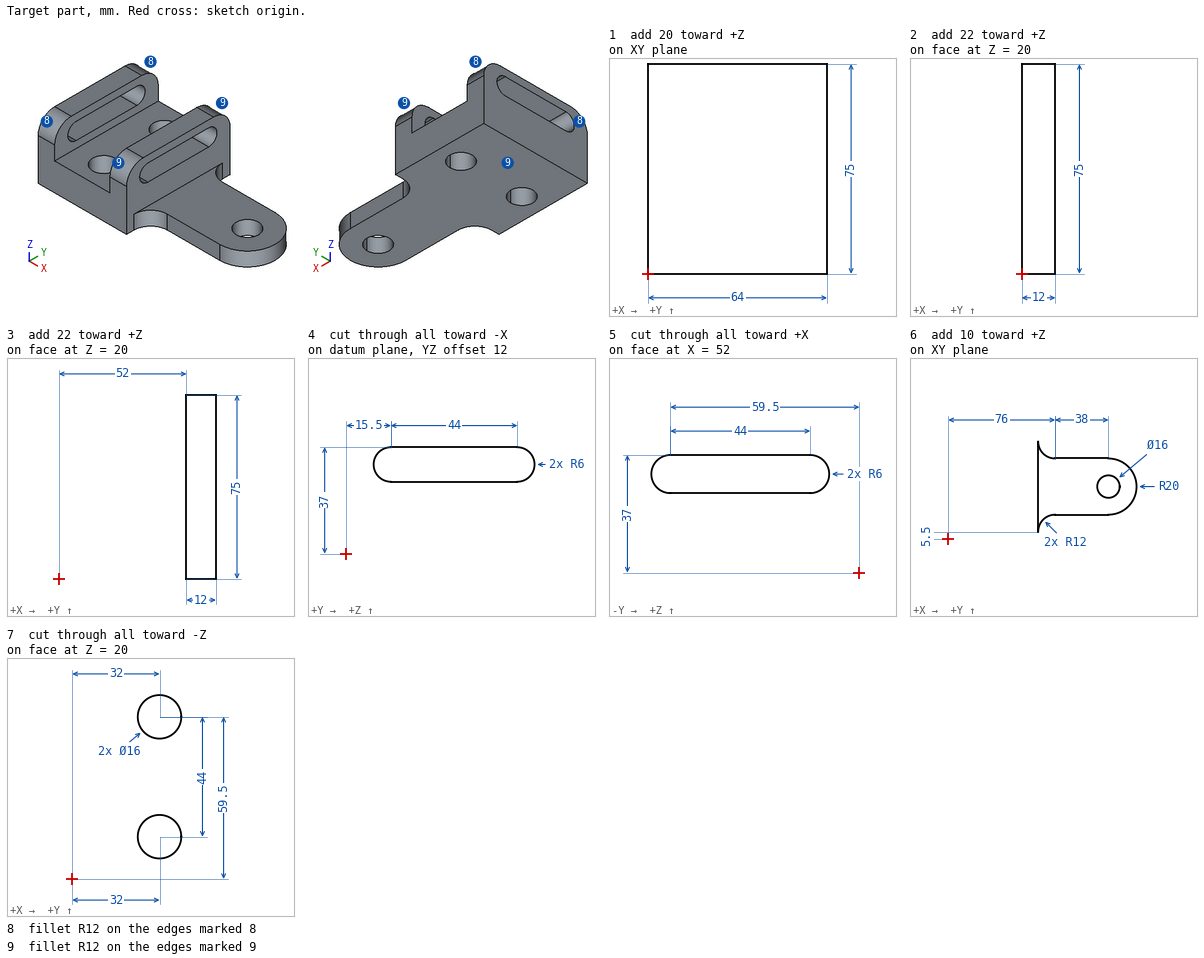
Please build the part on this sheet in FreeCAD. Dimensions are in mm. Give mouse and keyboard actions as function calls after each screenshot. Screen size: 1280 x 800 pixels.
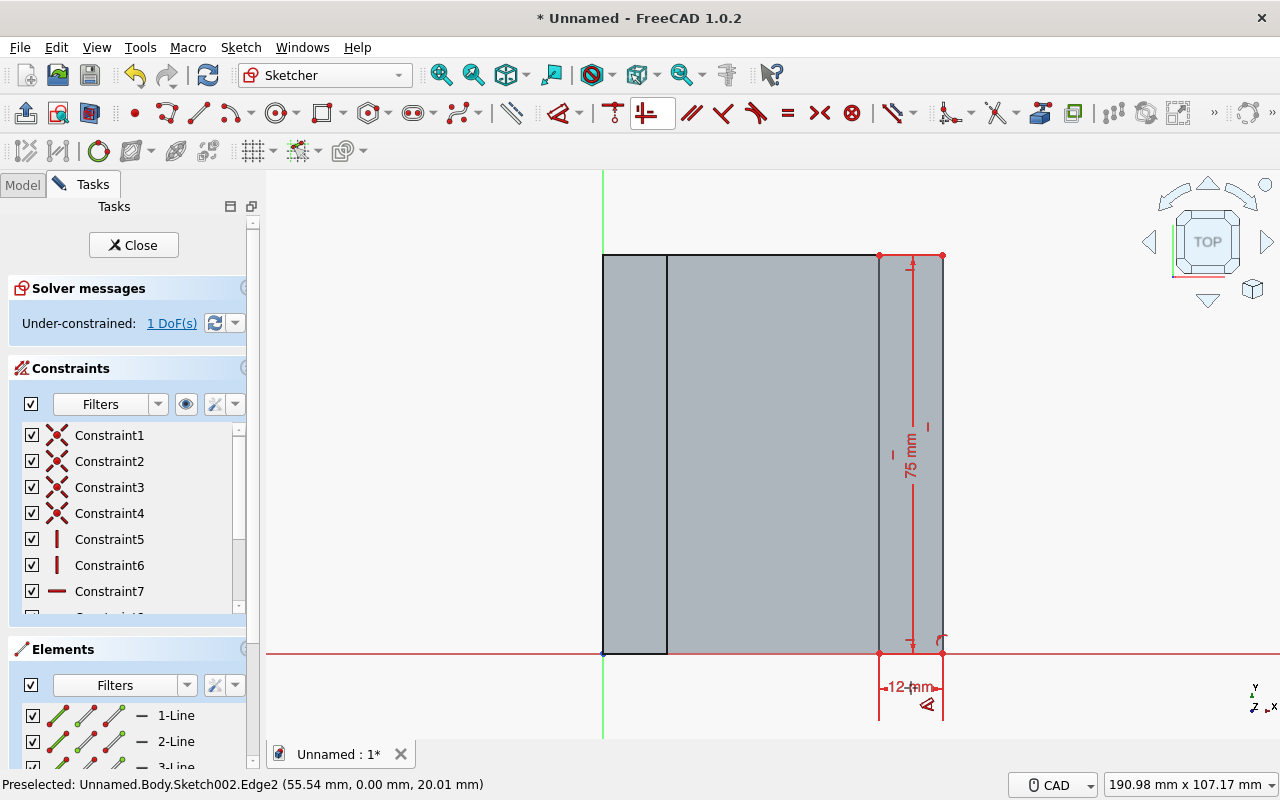
click(879, 255)
click(741, 688)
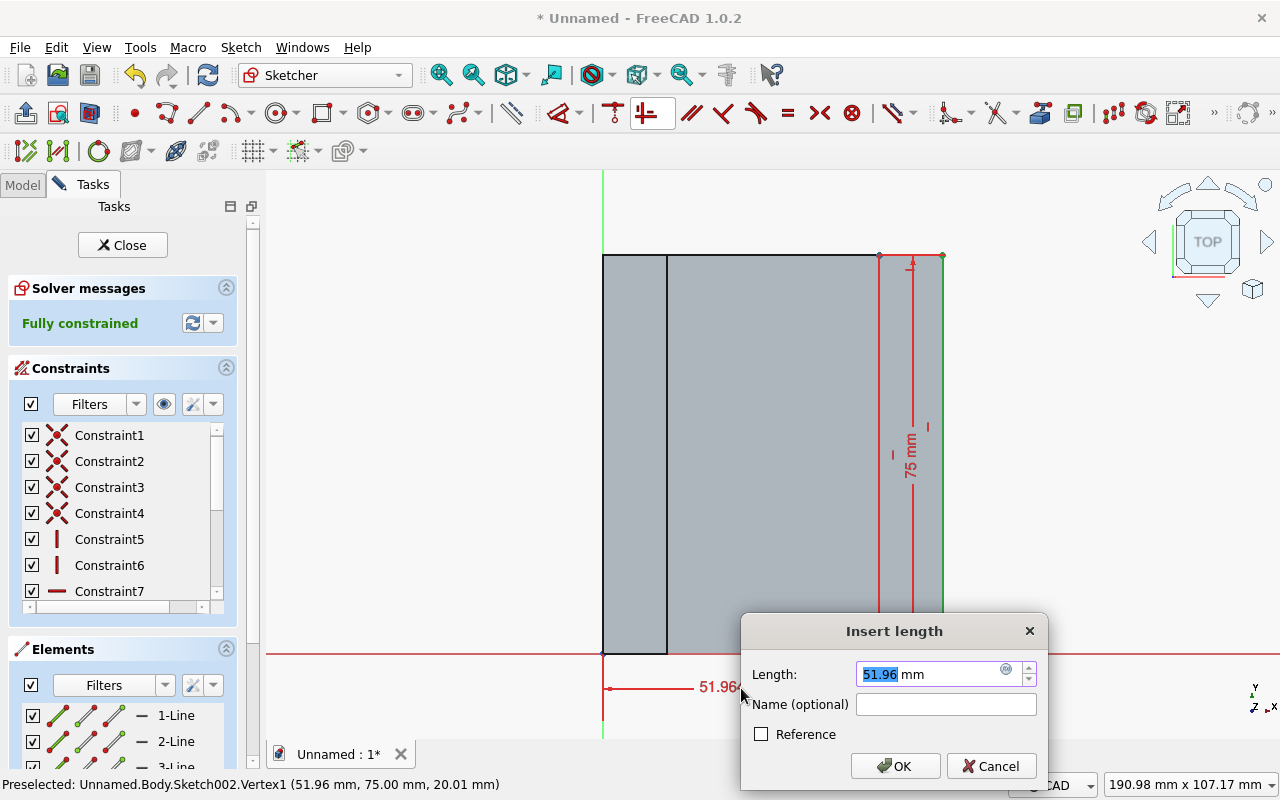
text(52)
key(Return)
key(Escape)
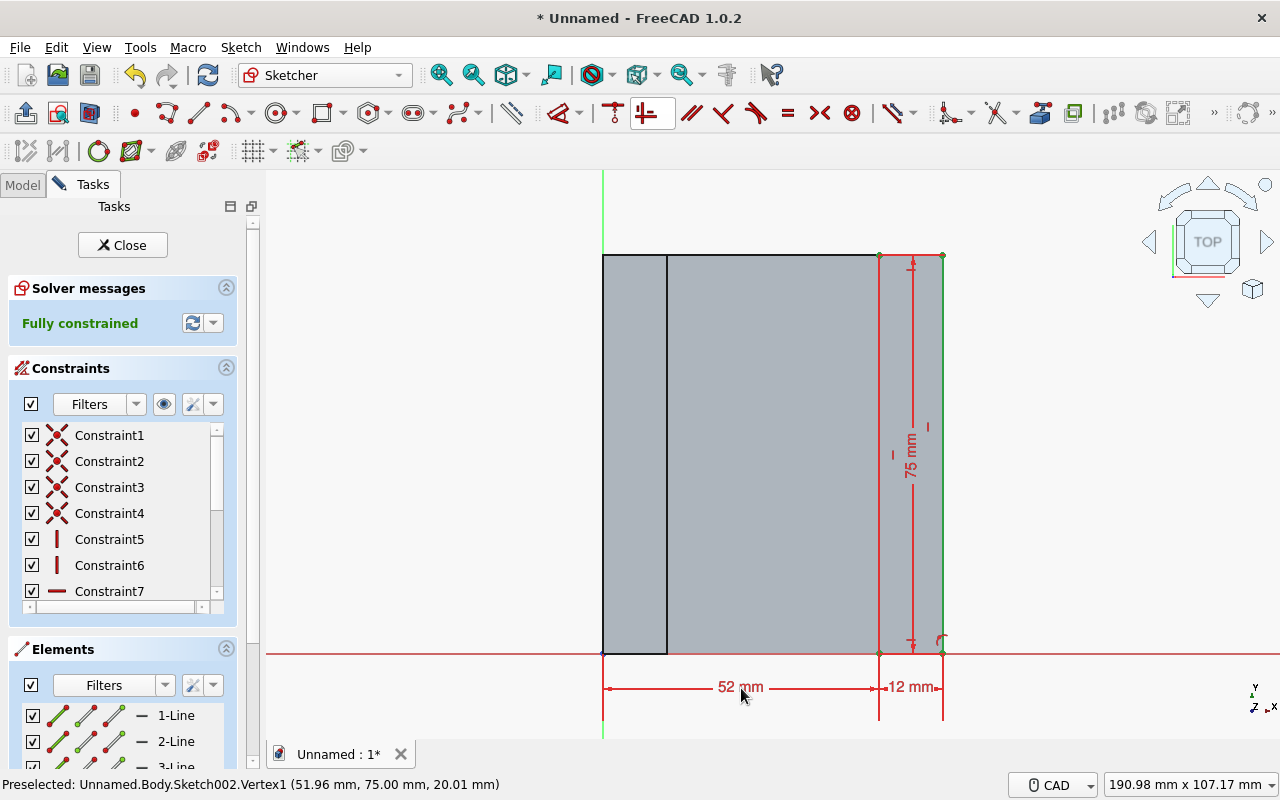
click(123, 245)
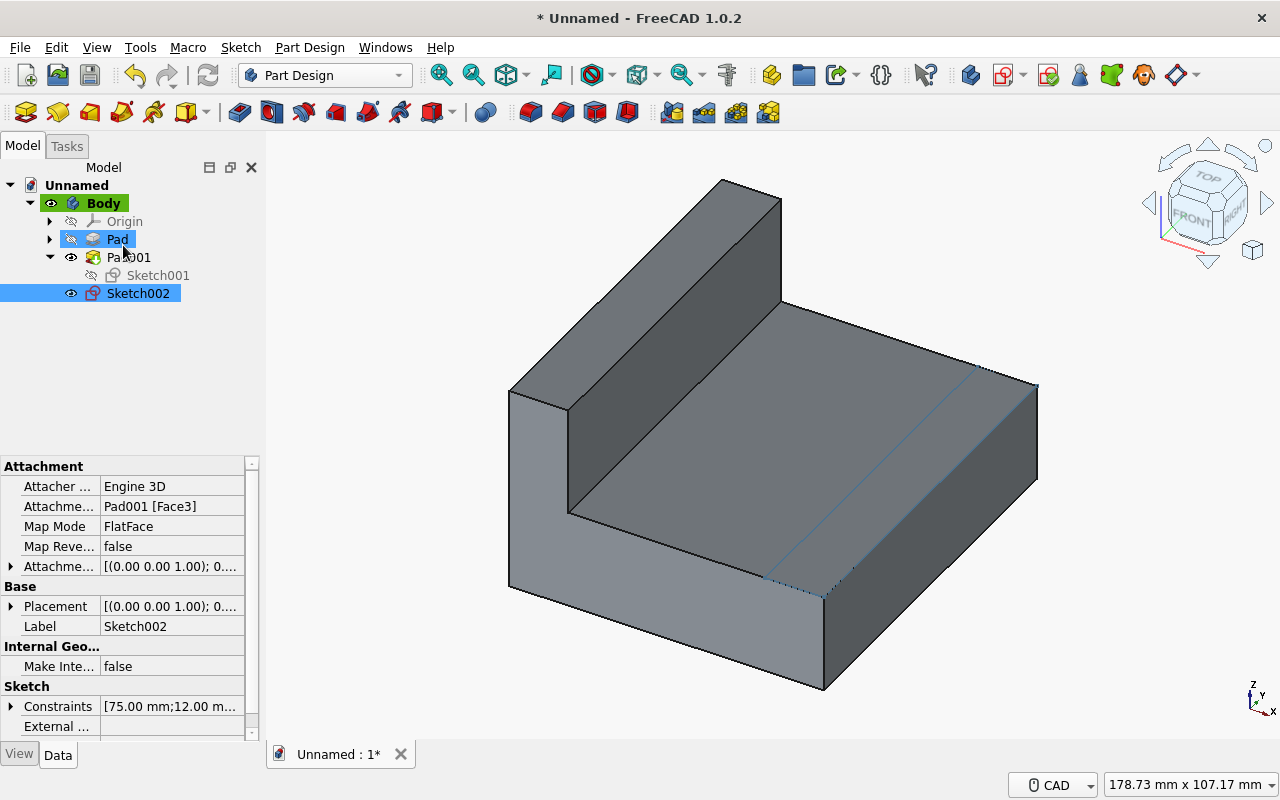
click(26, 112)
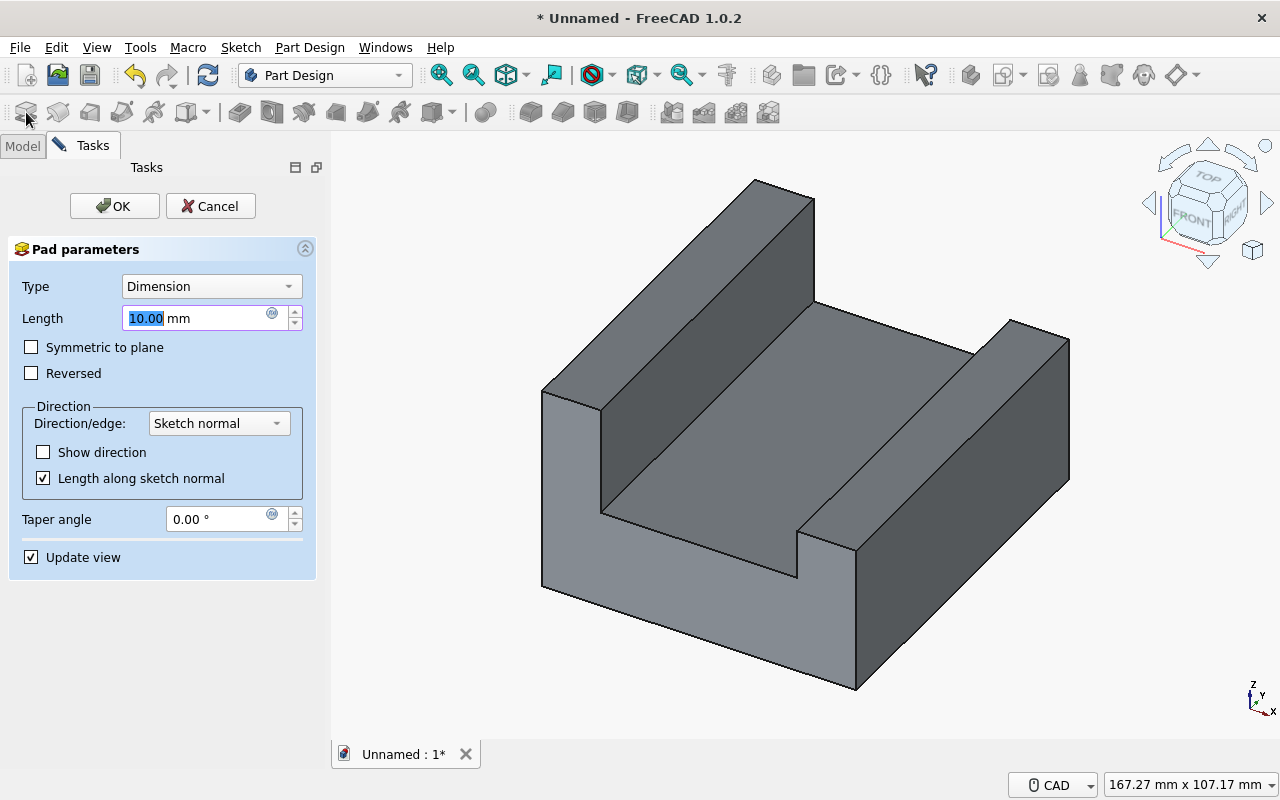
text(22)
key(Tab)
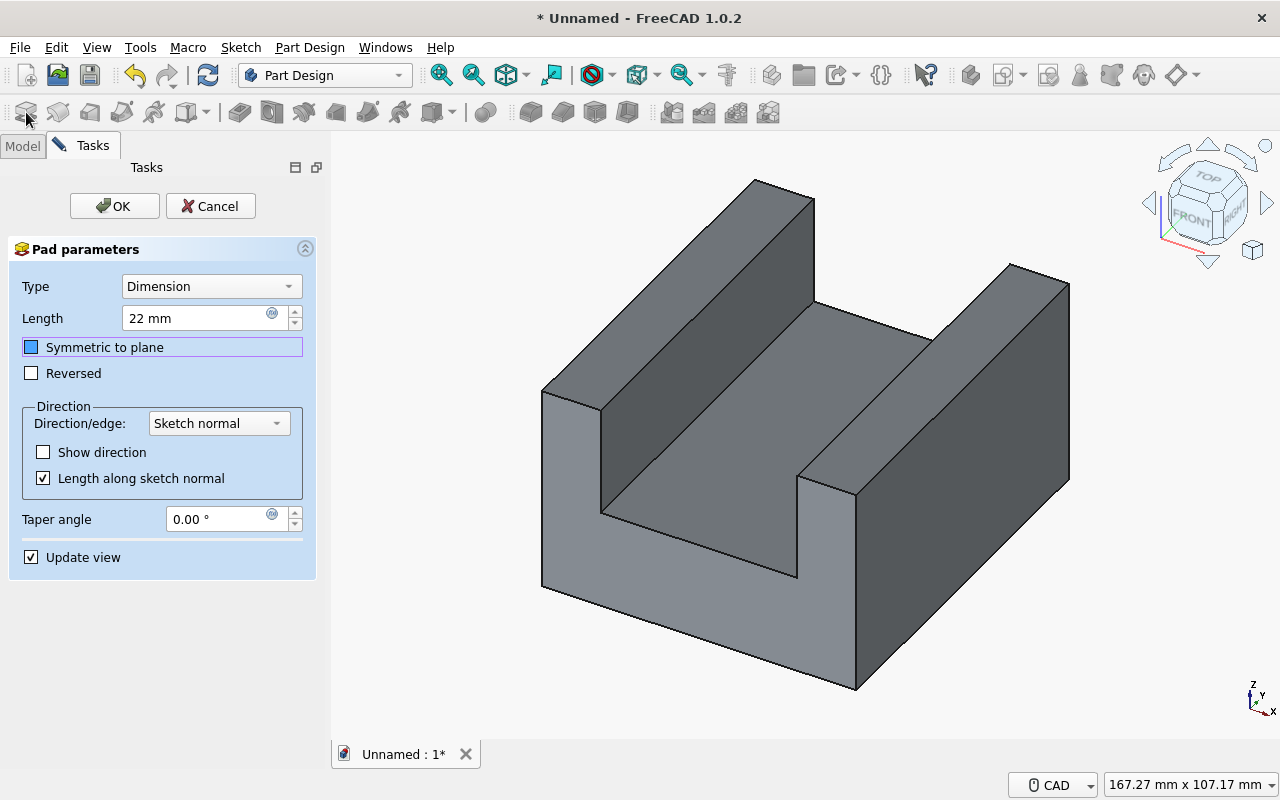
click(115, 206)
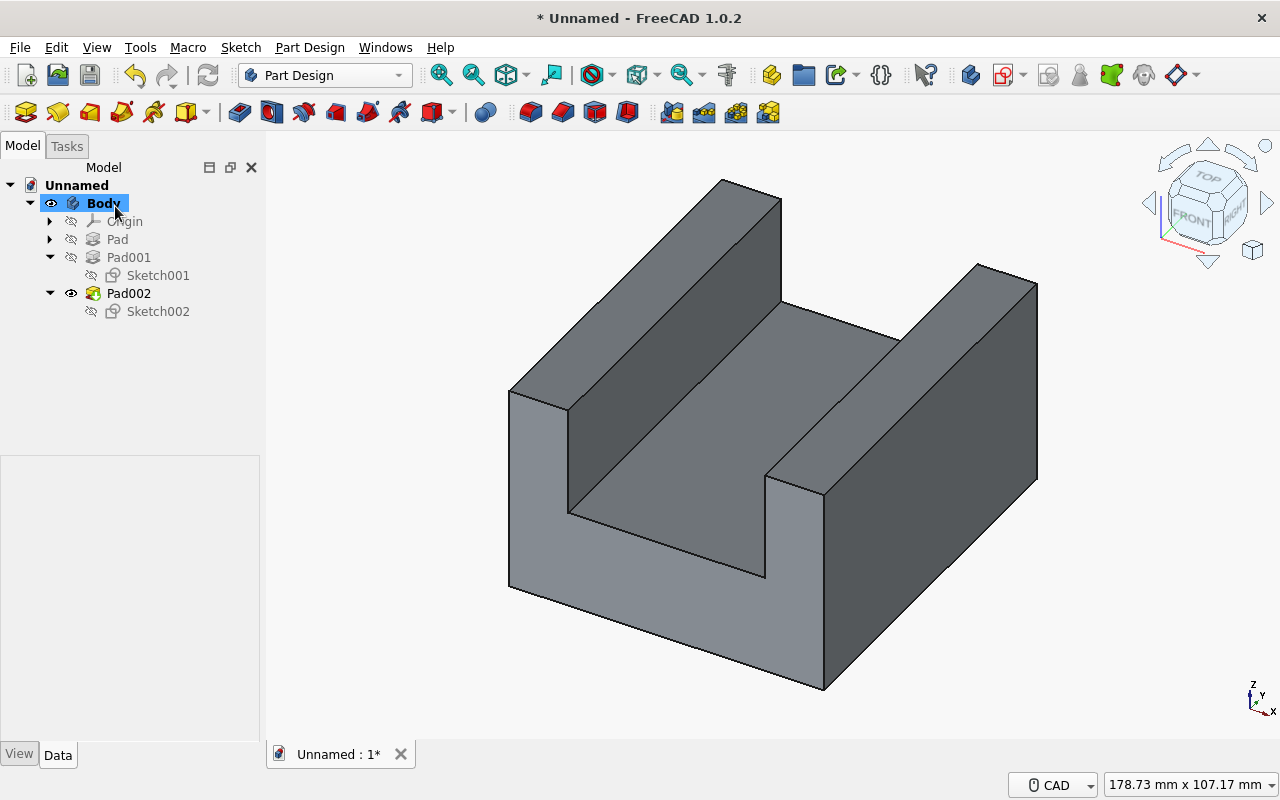
click(50, 221)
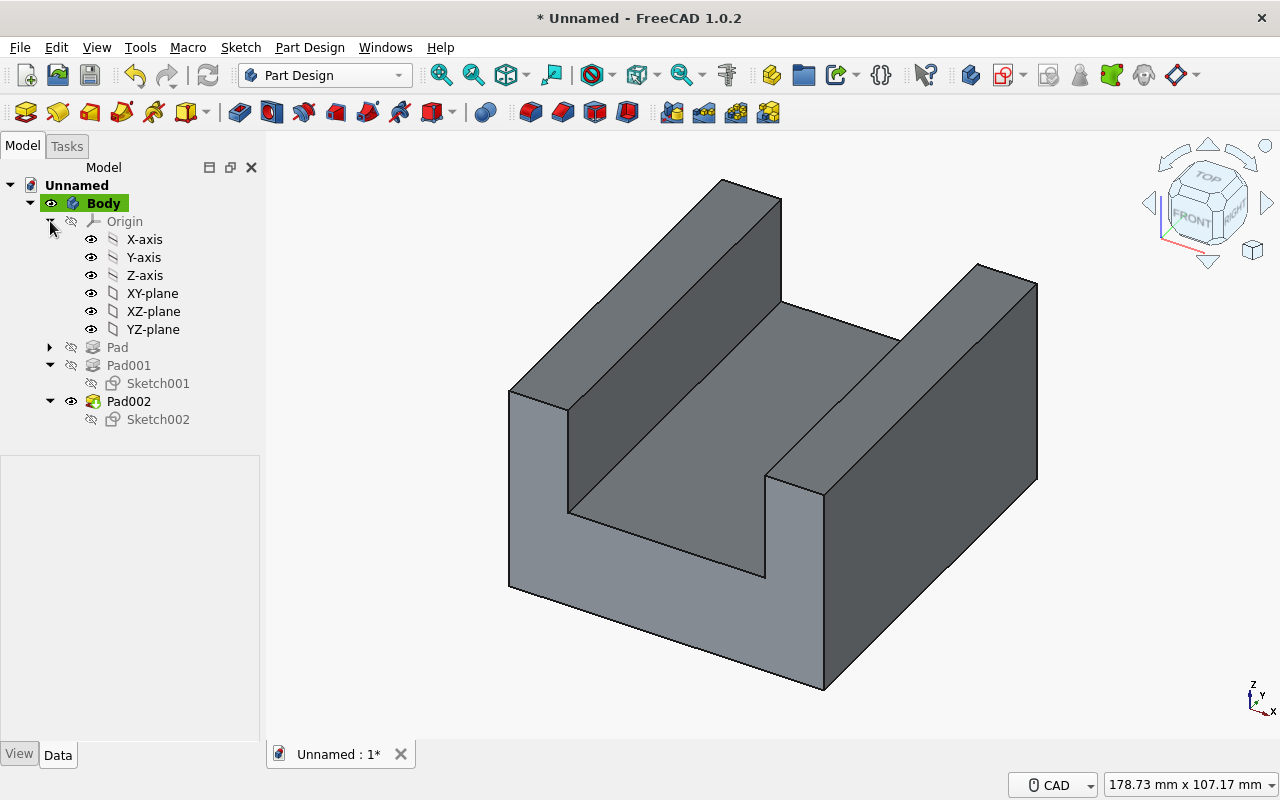
click(136, 329)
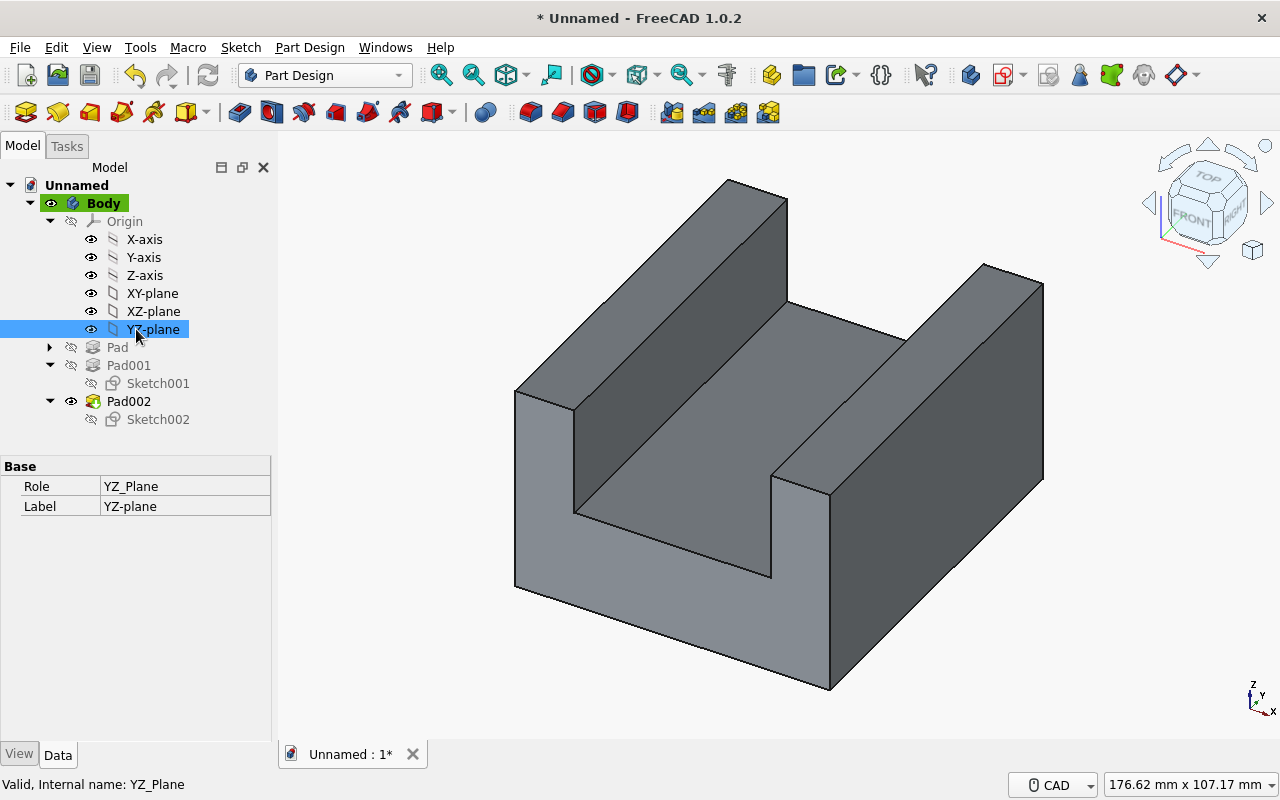
click(1176, 76)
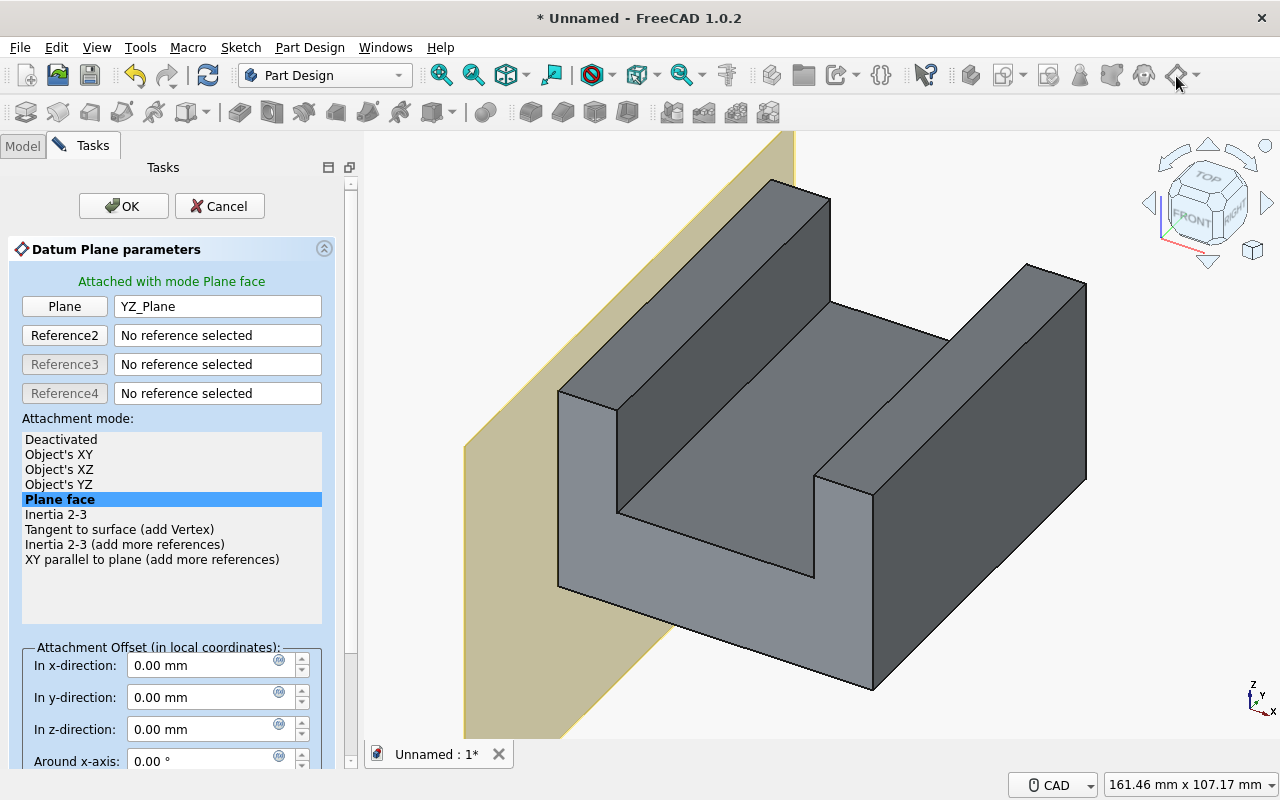
triple_click(210, 729)